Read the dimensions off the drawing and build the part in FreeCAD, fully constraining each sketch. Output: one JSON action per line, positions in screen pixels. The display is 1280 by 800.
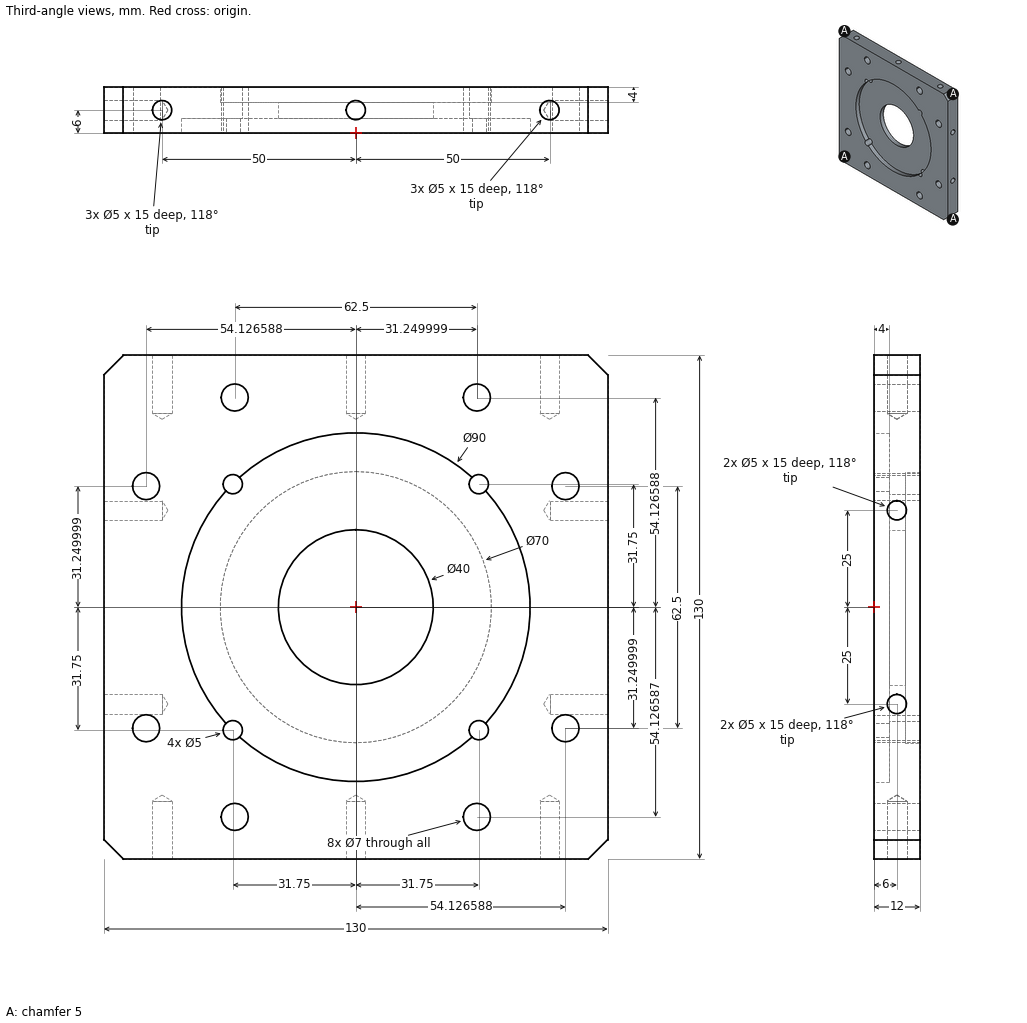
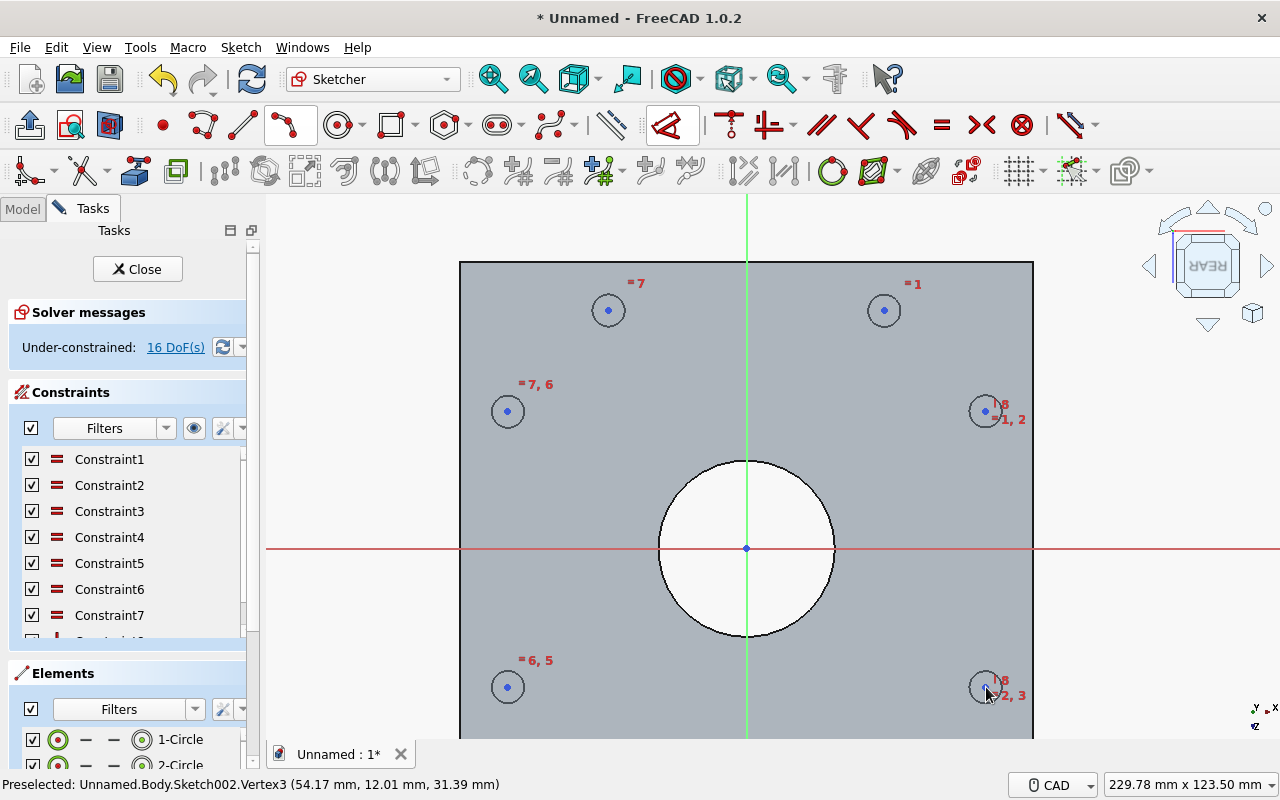
{"action": "scroll", "coordinate": [619, 299], "scroll_direction": "down", "scroll_amount": 2}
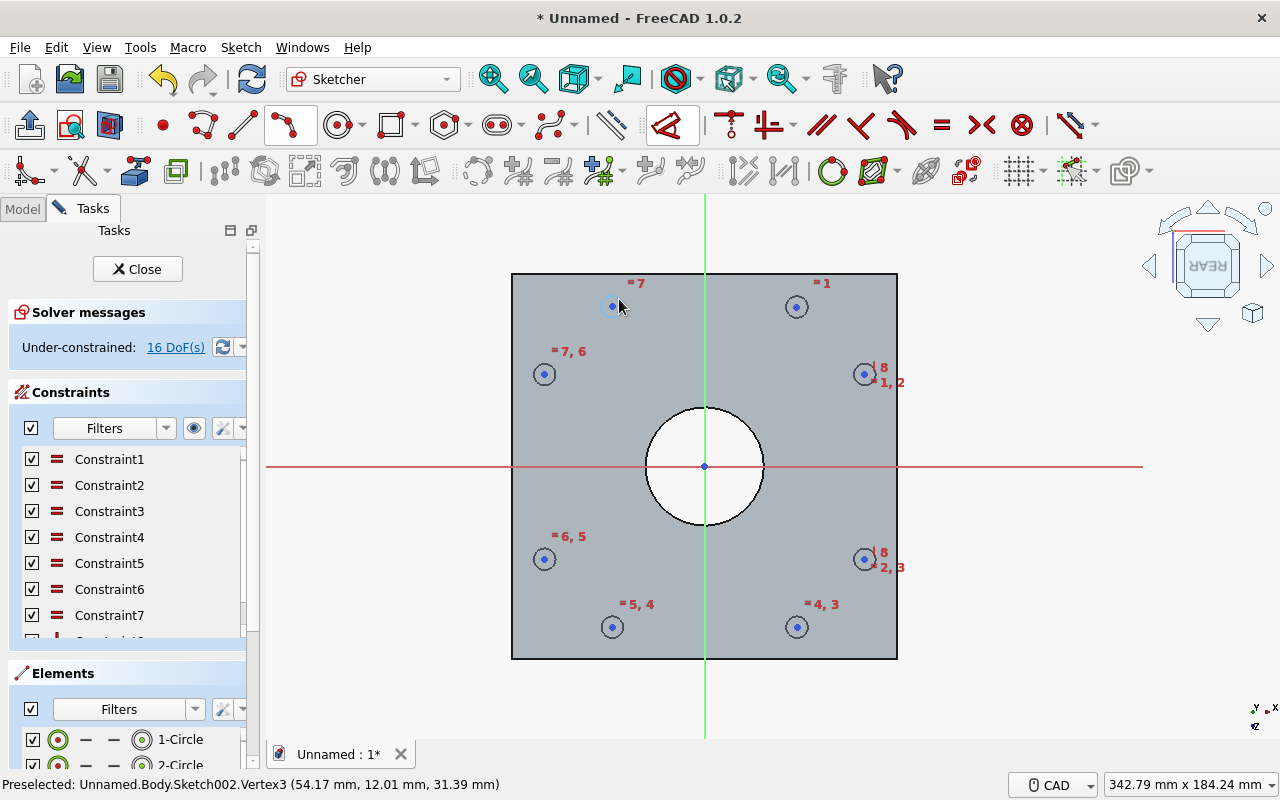
{"action": "left_click", "coordinate": [797, 627]}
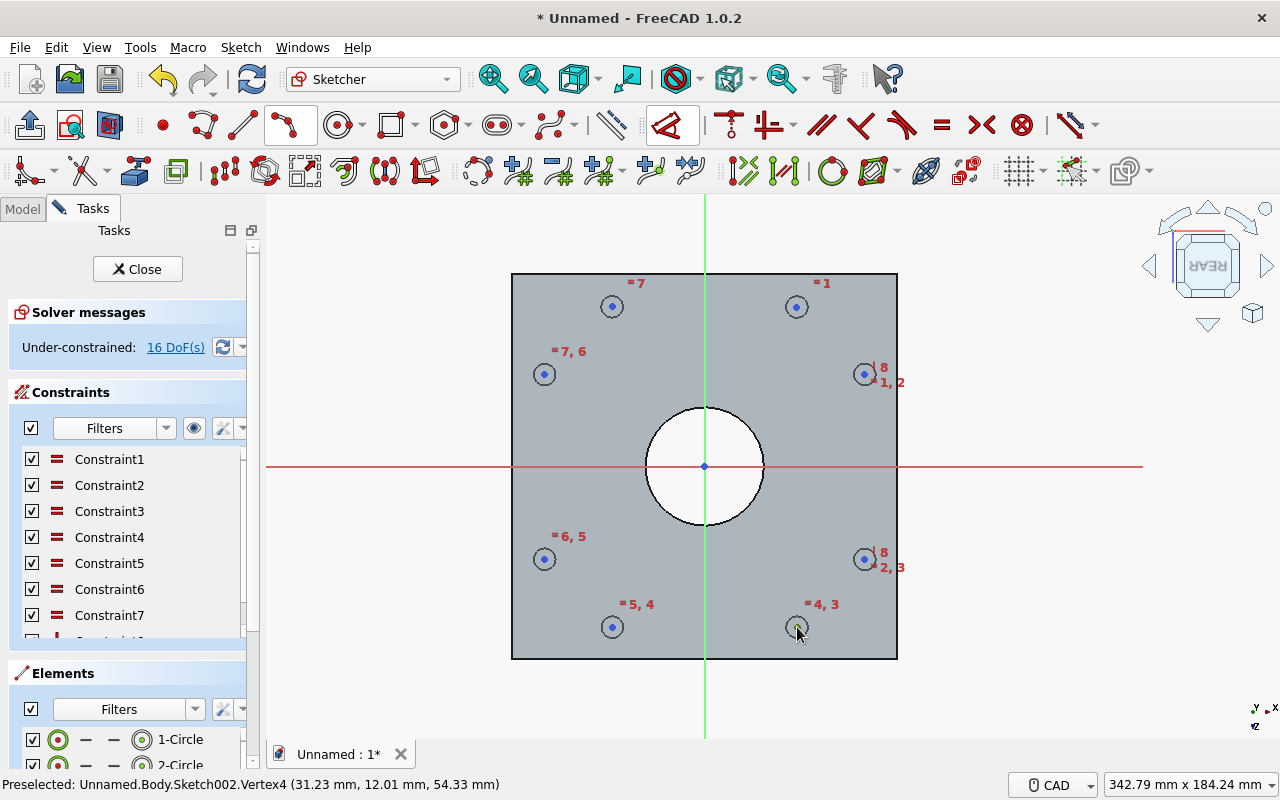
{"action": "left_click", "coordinate": [612, 627]}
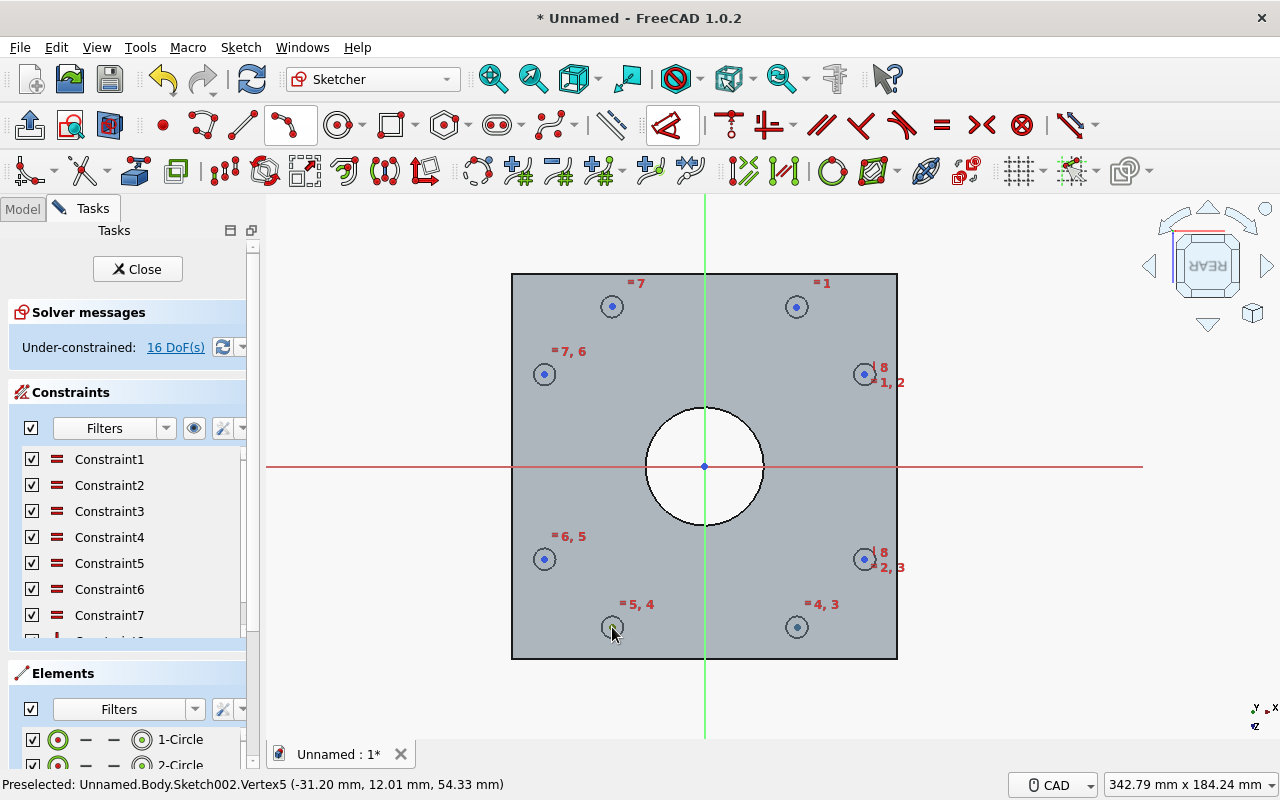
{"action": "key", "text": "h"}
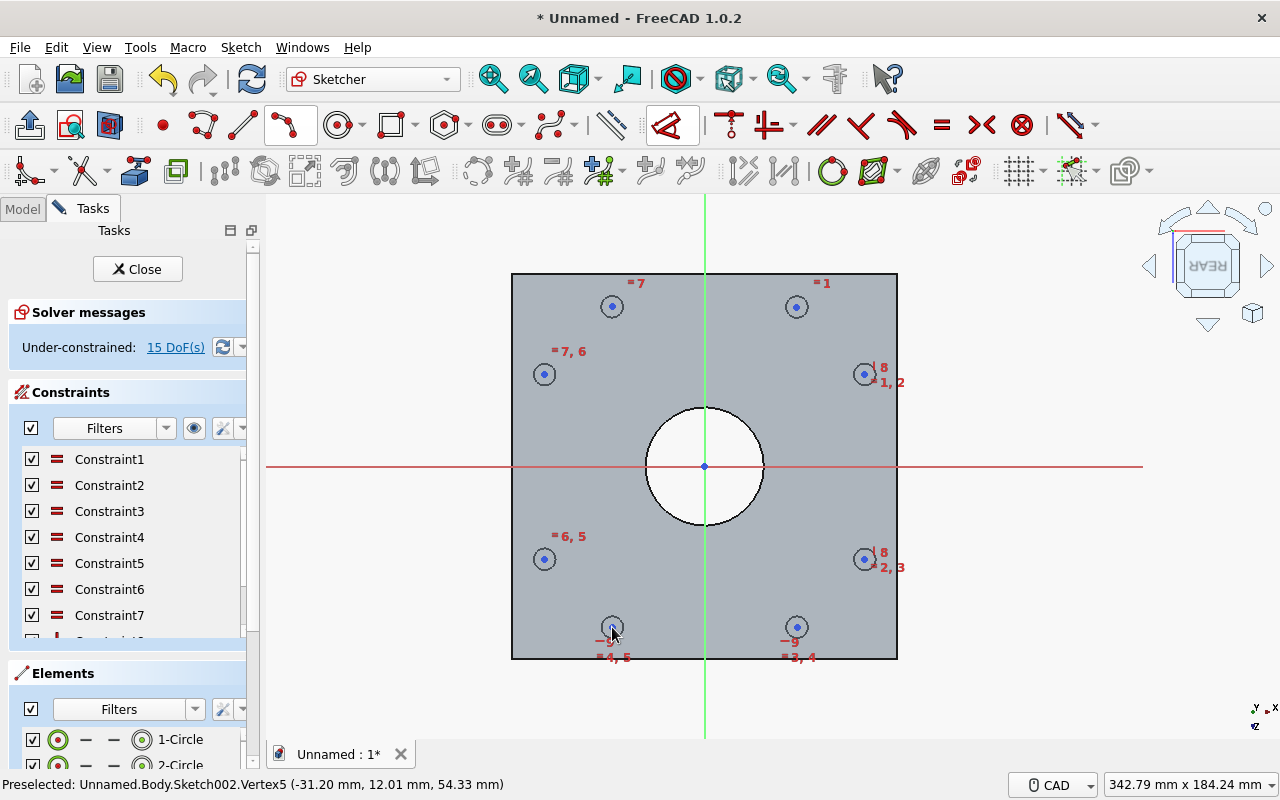
{"action": "left_click", "coordinate": [545, 559]}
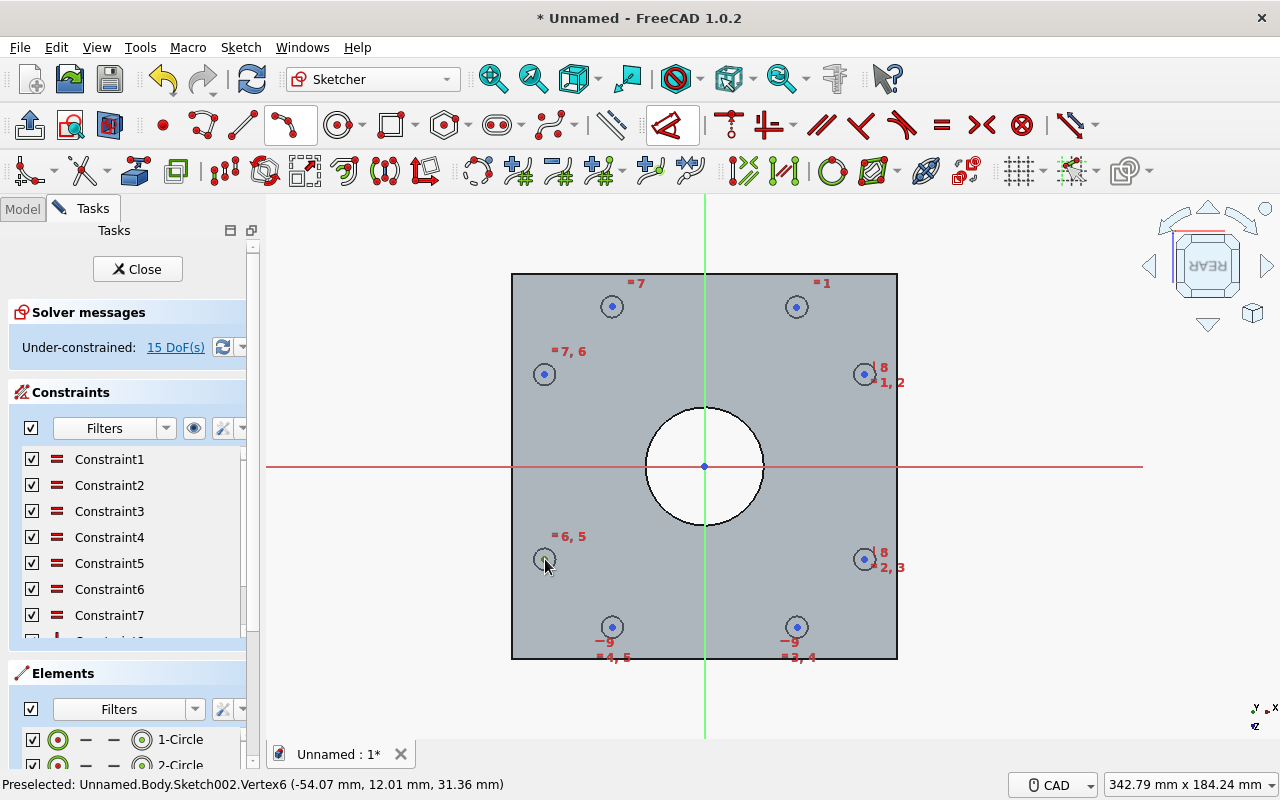
{"action": "left_click", "coordinate": [545, 375]}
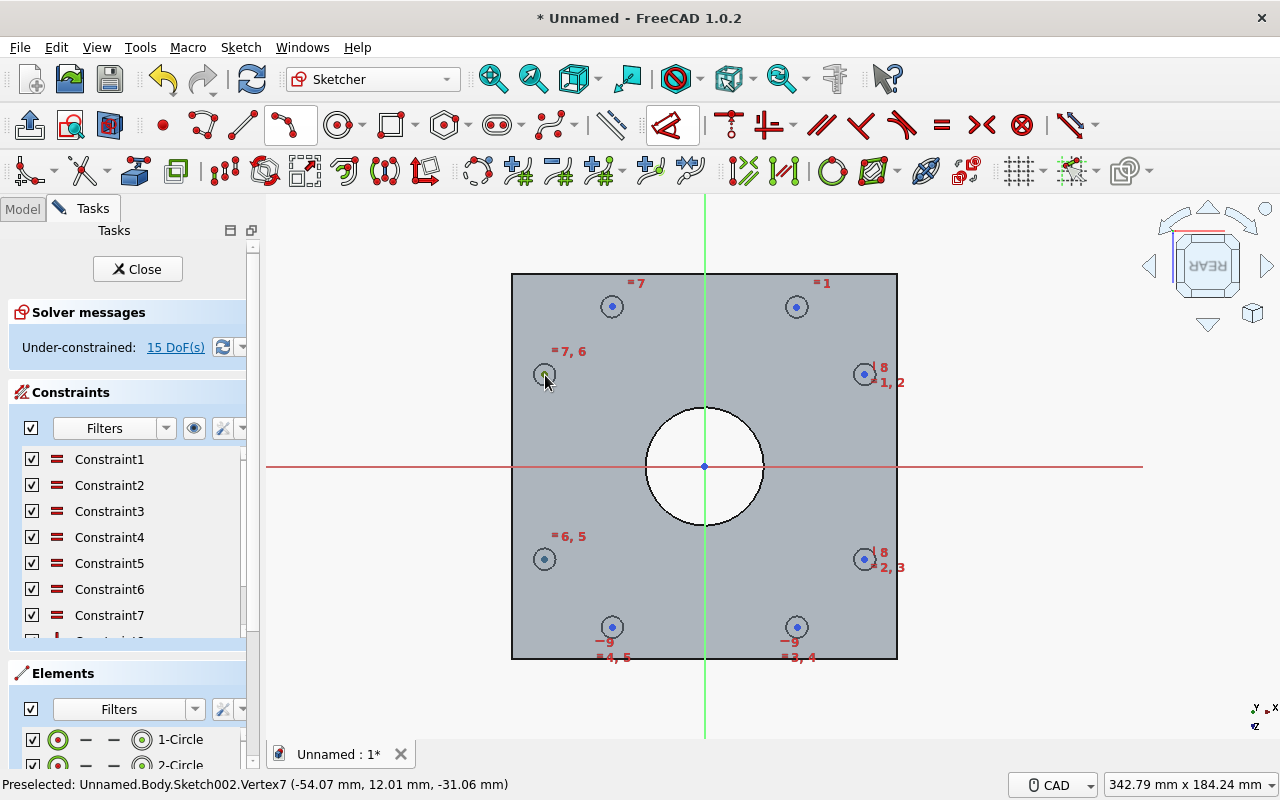
{"action": "left_click", "coordinate": [796, 126]}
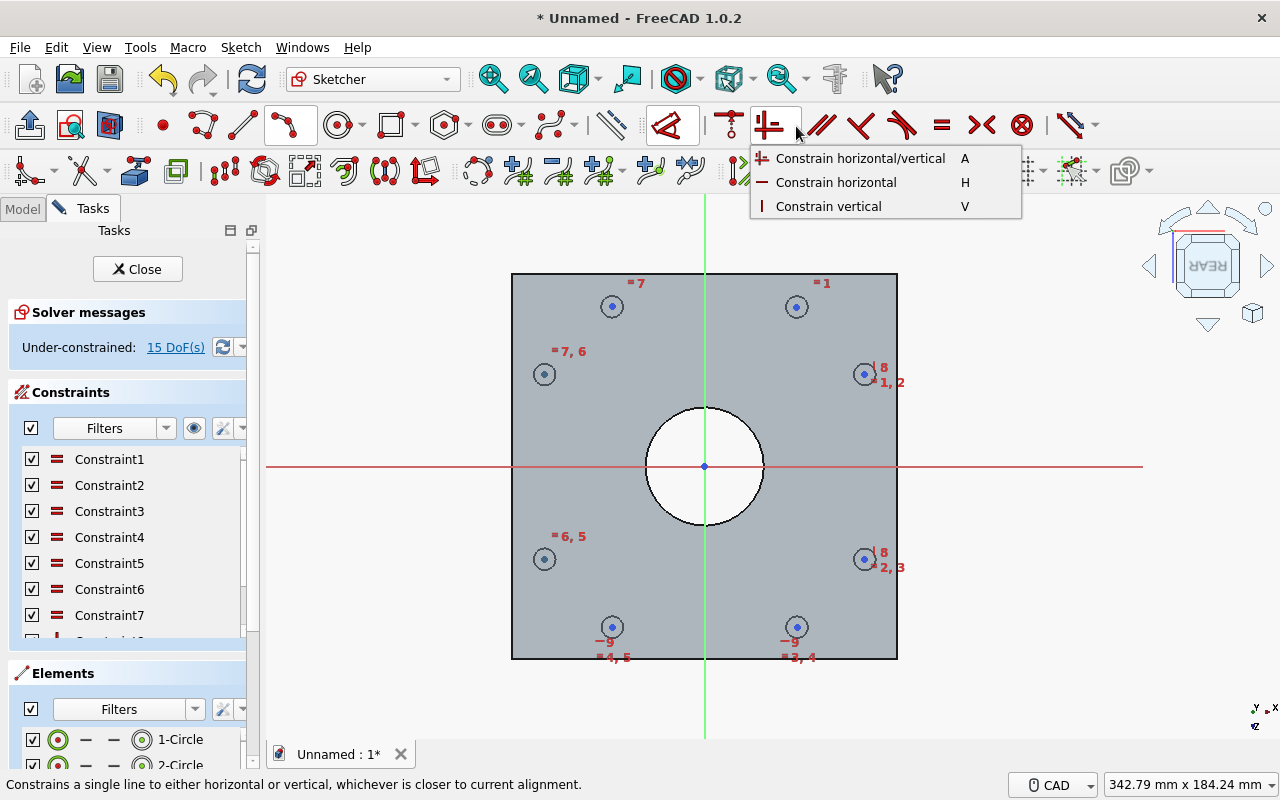
{"action": "left_click", "coordinate": [886, 206]}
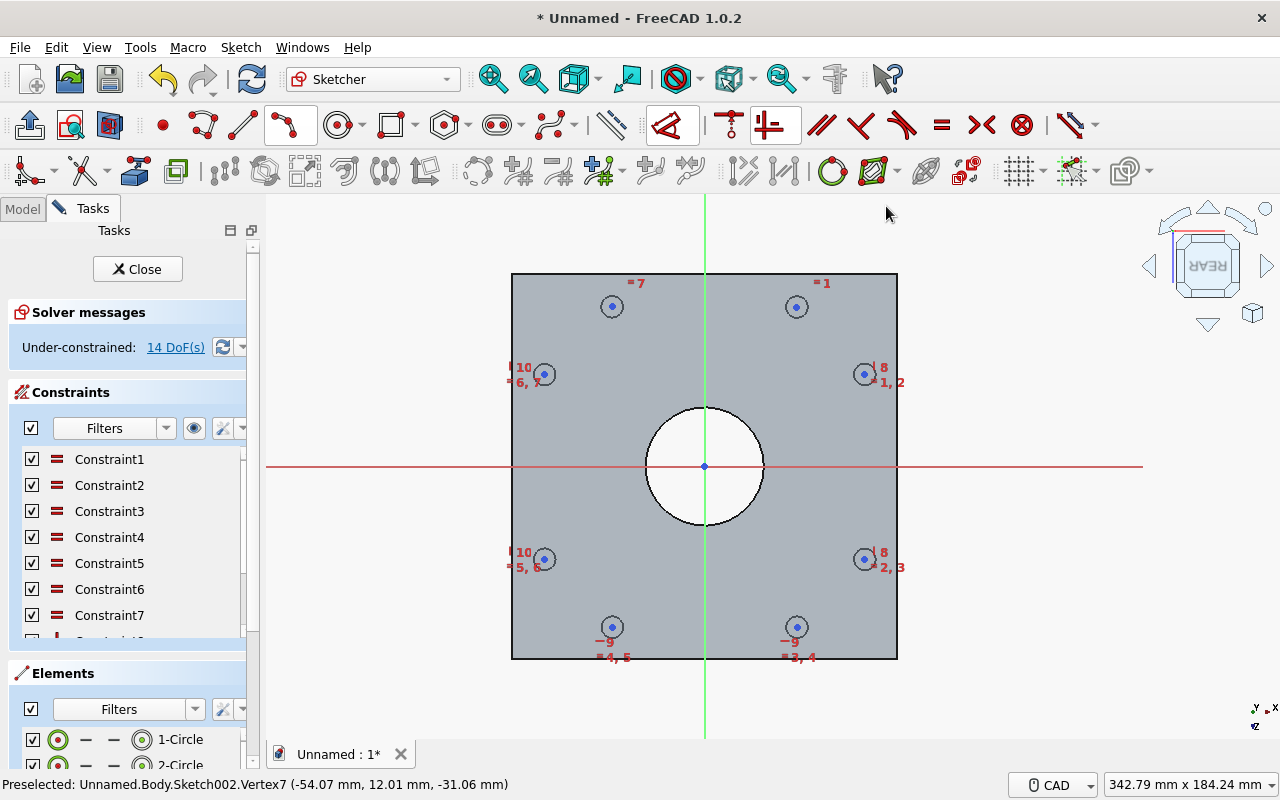
{"action": "left_click", "coordinate": [797, 307]}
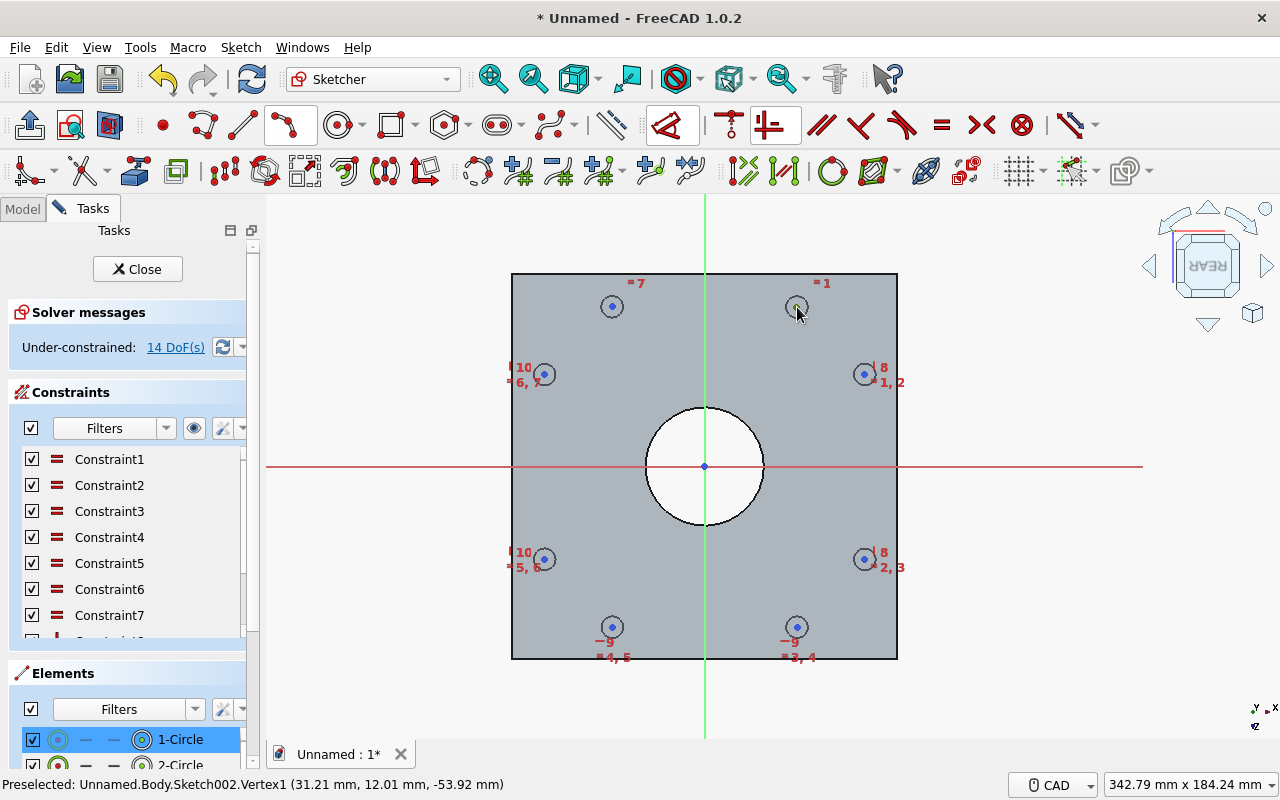
{"action": "left_click", "coordinate": [612, 307]}